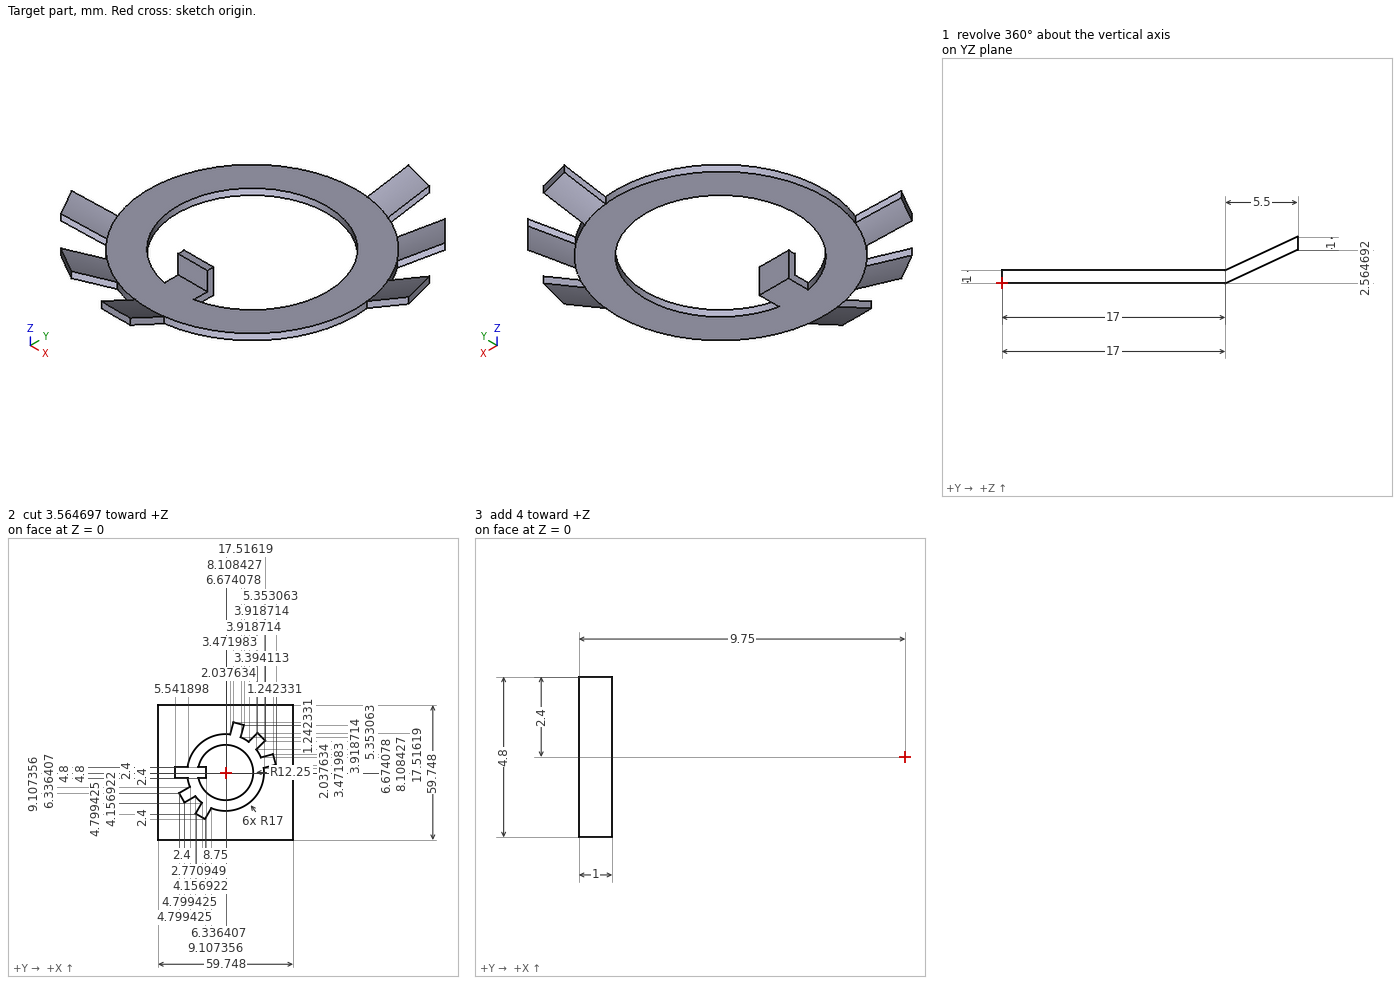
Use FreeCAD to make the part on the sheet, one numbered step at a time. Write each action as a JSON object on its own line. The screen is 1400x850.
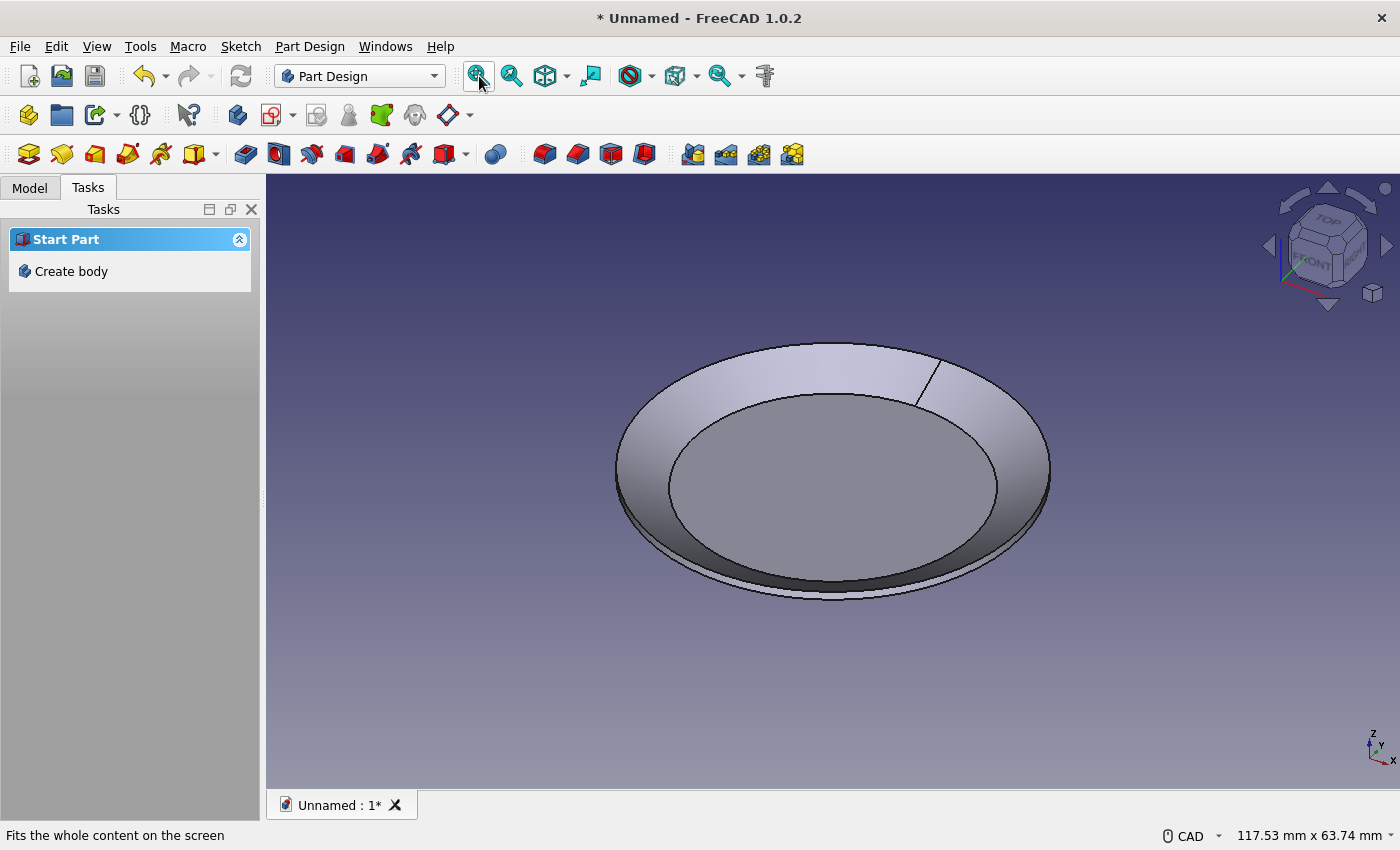
{"action": "key", "text": "5"}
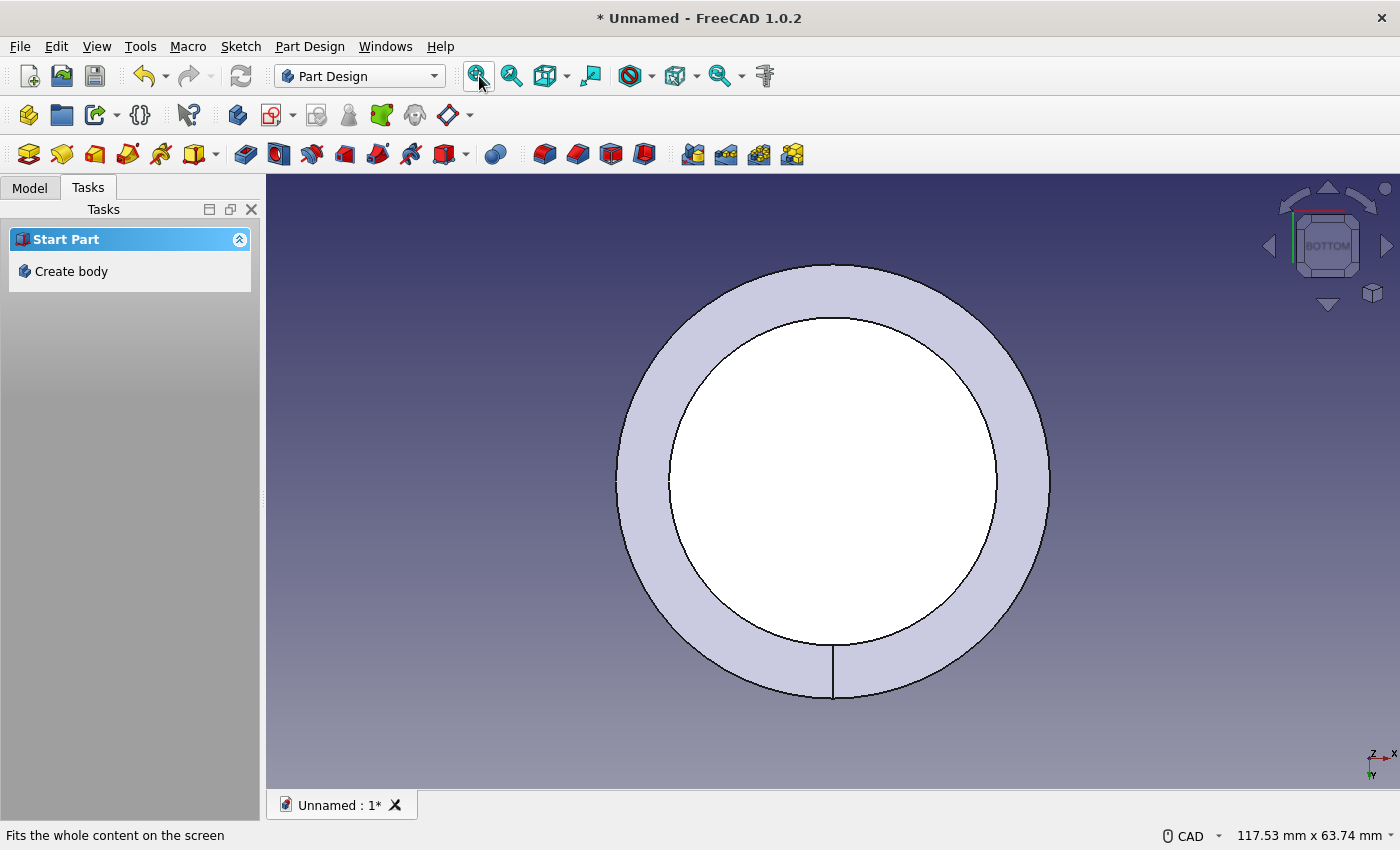
{"action": "left_click", "coordinate": [833, 480]}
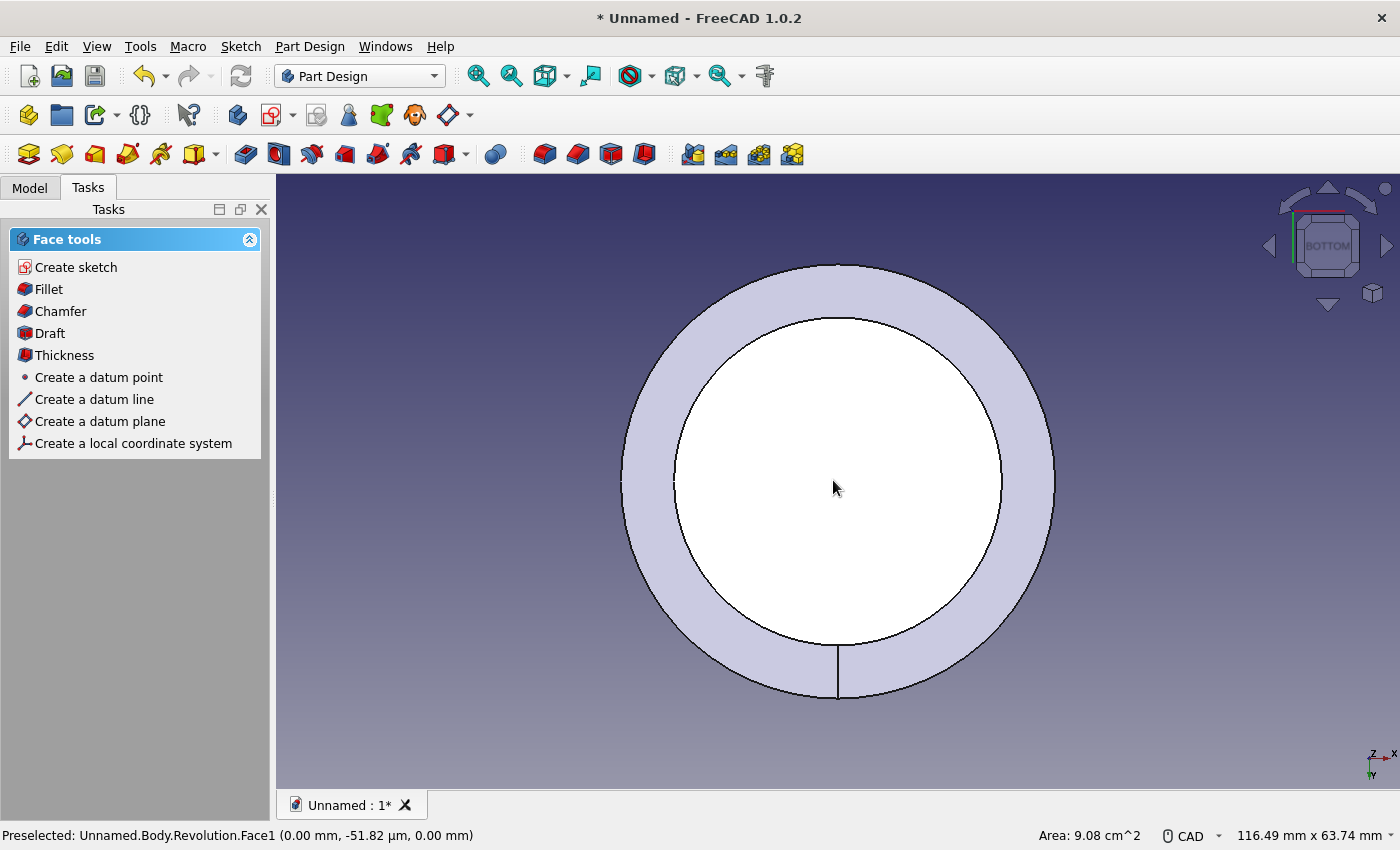
{"action": "left_click", "coordinate": [270, 116]}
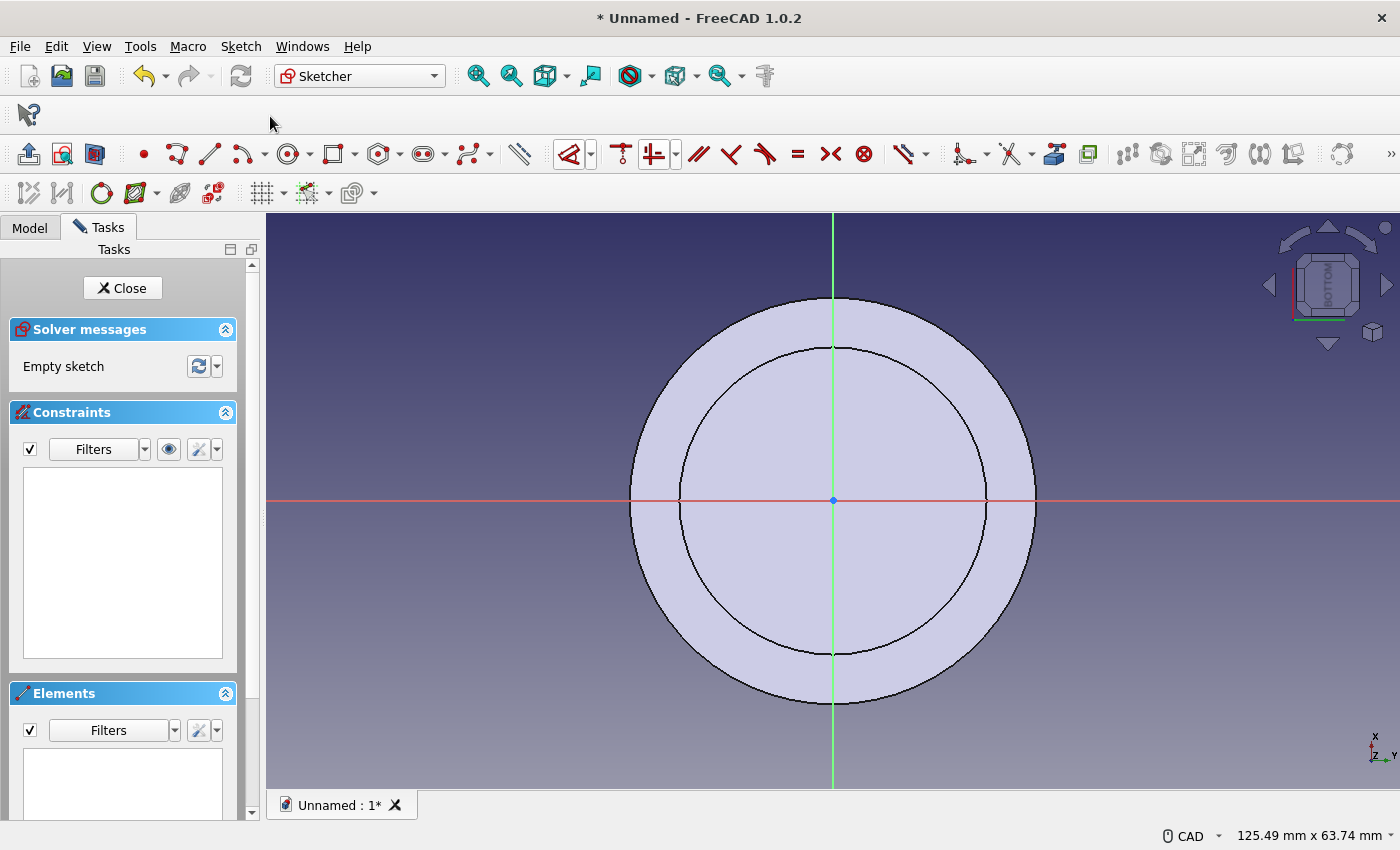
{"action": "scroll", "coordinate": [625, 501], "scroll_direction": "down", "scroll_amount": 2}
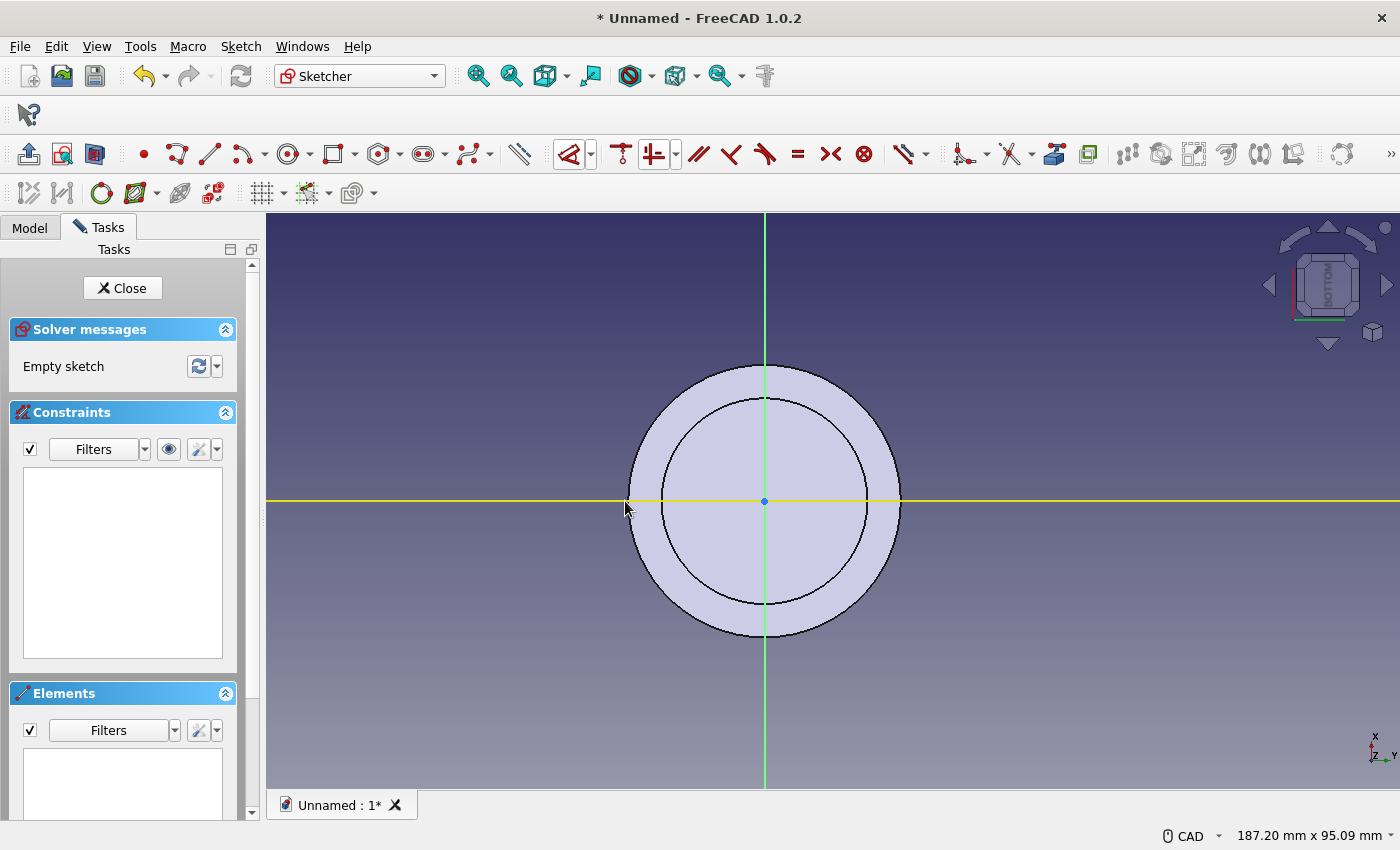
{"action": "left_click", "coordinate": [354, 154]}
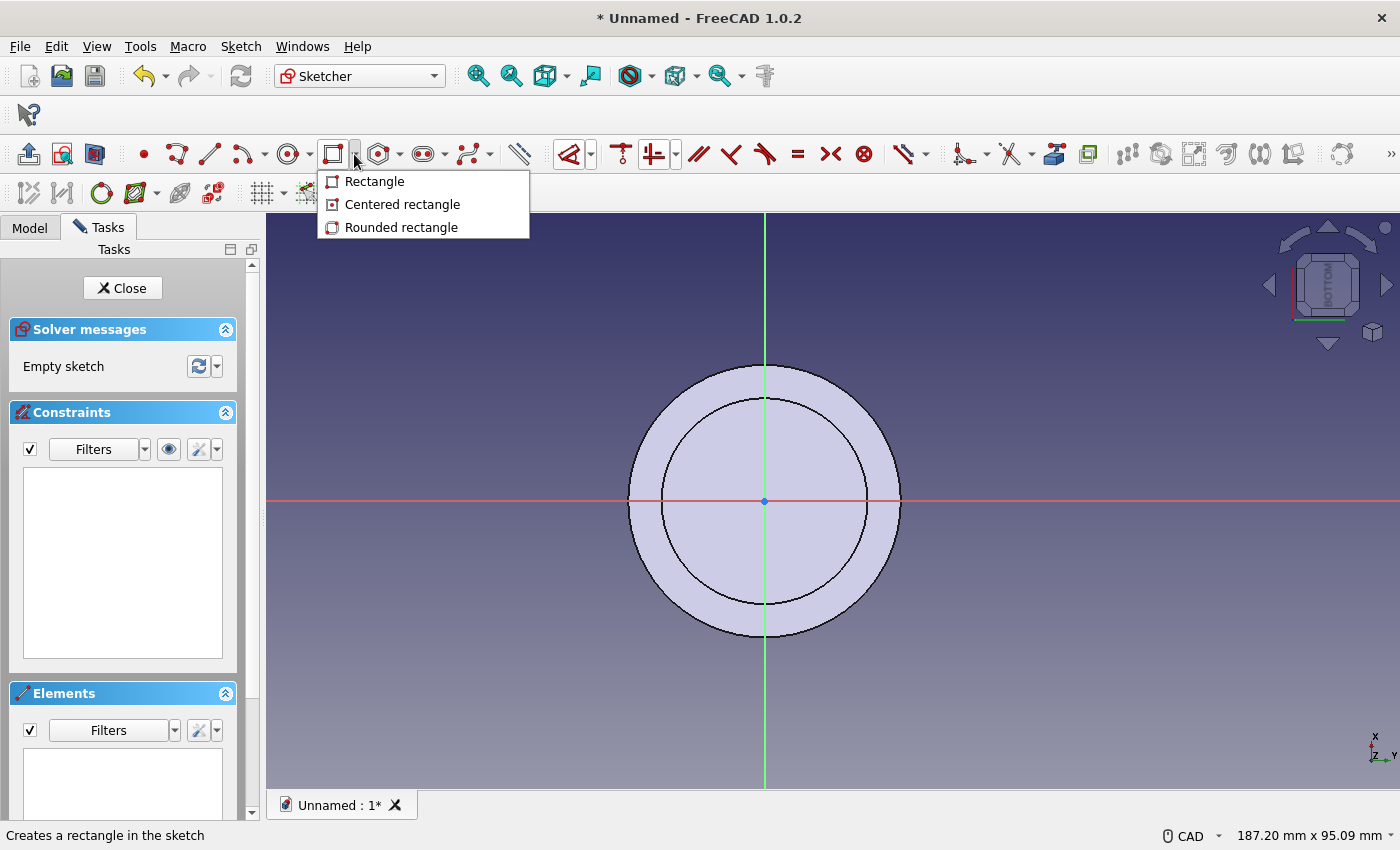
{"action": "left_click", "coordinate": [424, 204]}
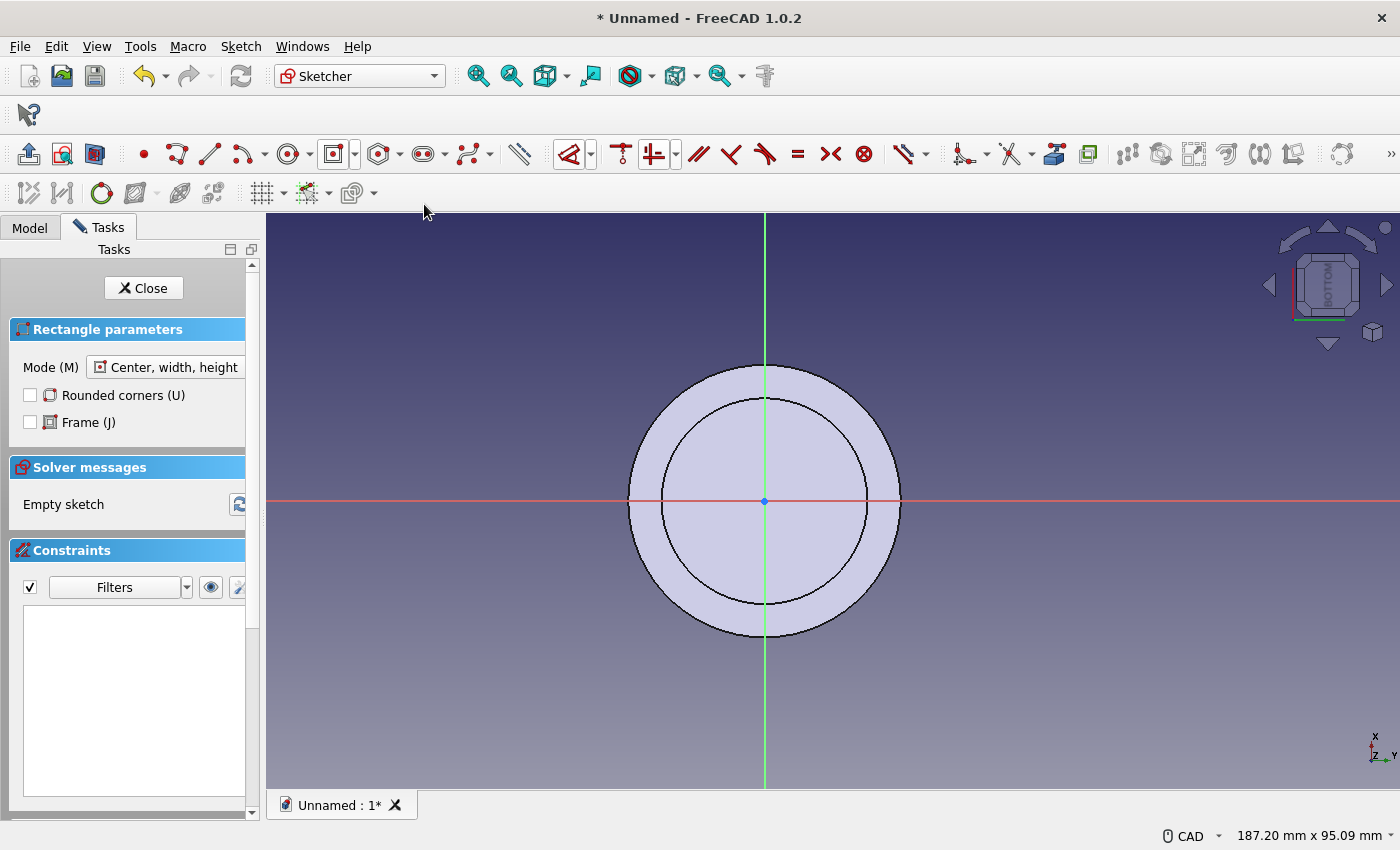
{"action": "left_click", "coordinate": [765, 501]}
{"action": "mouse_move", "coordinate": [945, 320]}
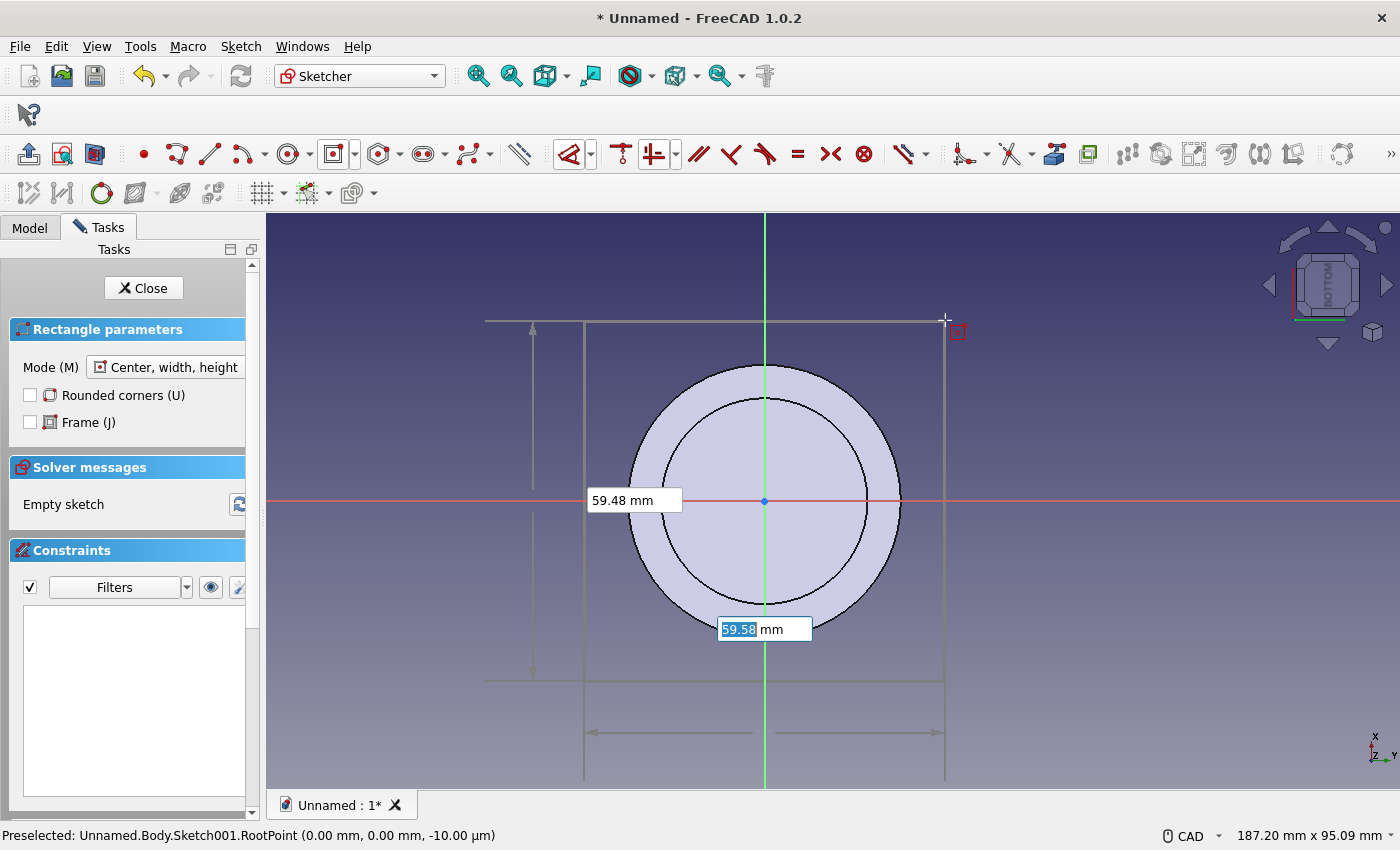
{"action": "type", "text": "59.748"}
{"action": "key", "text": "Tab"}
{"action": "type", "text": "59.748"}
{"action": "key", "text": "Return"}